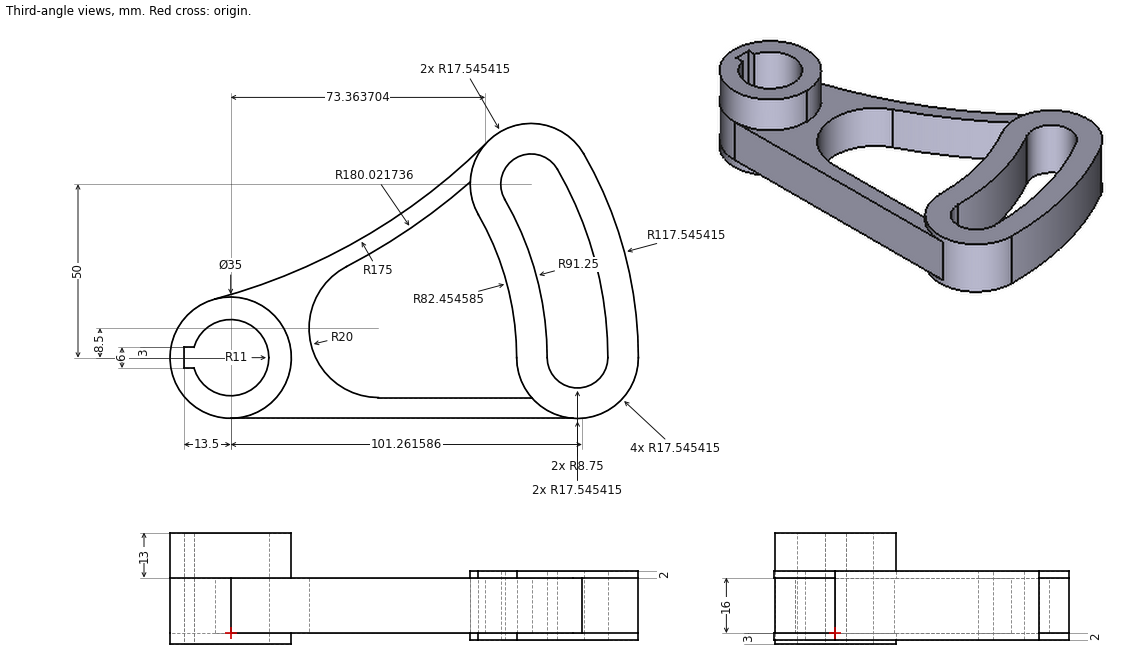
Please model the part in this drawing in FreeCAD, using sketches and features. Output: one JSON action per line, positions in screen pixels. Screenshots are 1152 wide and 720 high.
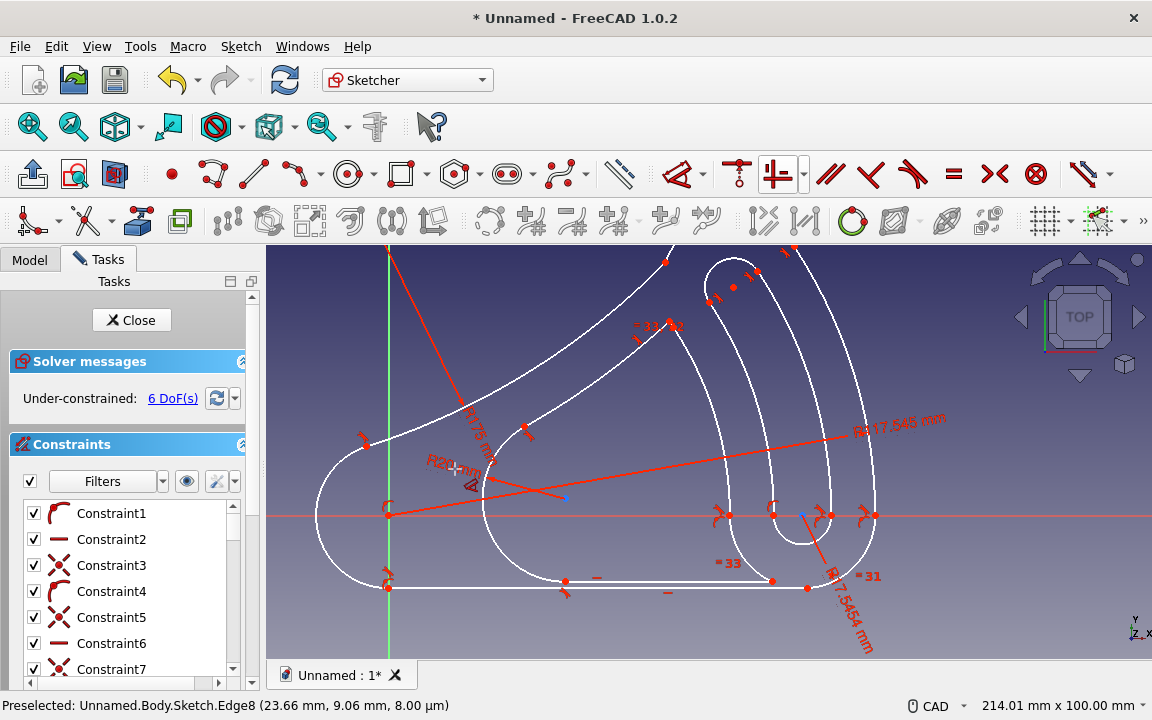
{"action": "left_click", "coordinate": [571, 399]}
{"action": "left_click", "coordinate": [589, 426]}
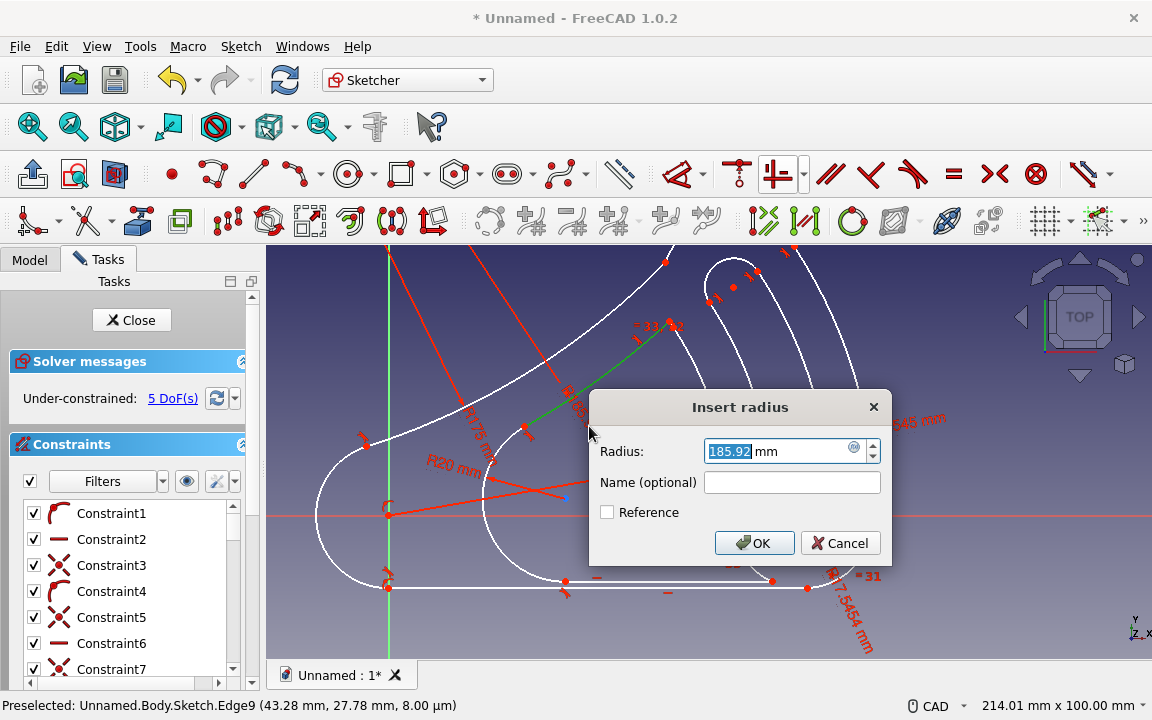
{"action": "type", "text": "180.021736"}
{"action": "key", "text": "Return"}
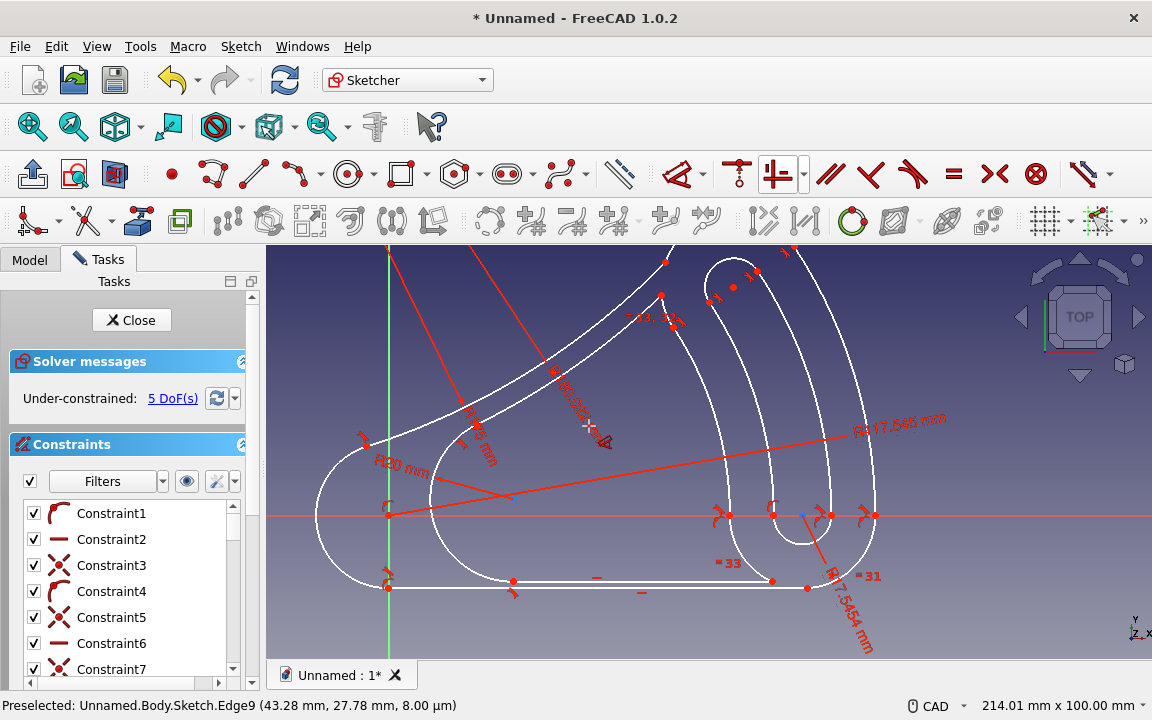
{"action": "left_click", "coordinate": [707, 277]}
{"action": "left_click", "coordinate": [712, 344]}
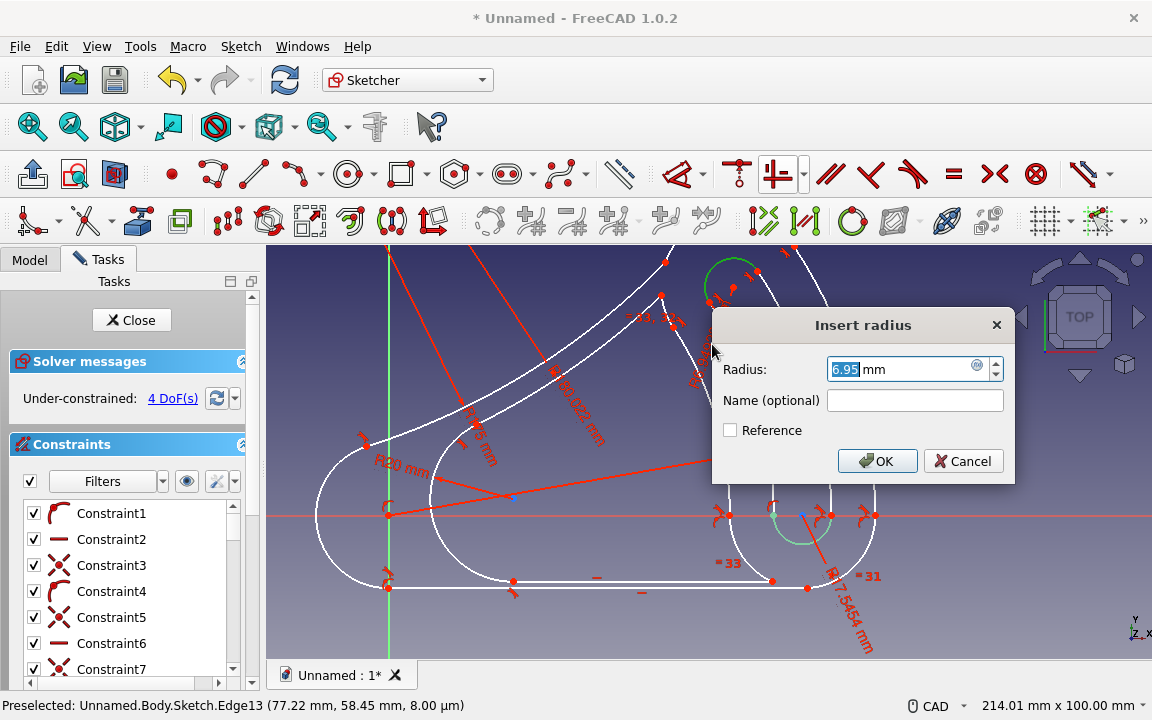
{"action": "type", "text": "8.75"}
{"action": "key", "text": "Return"}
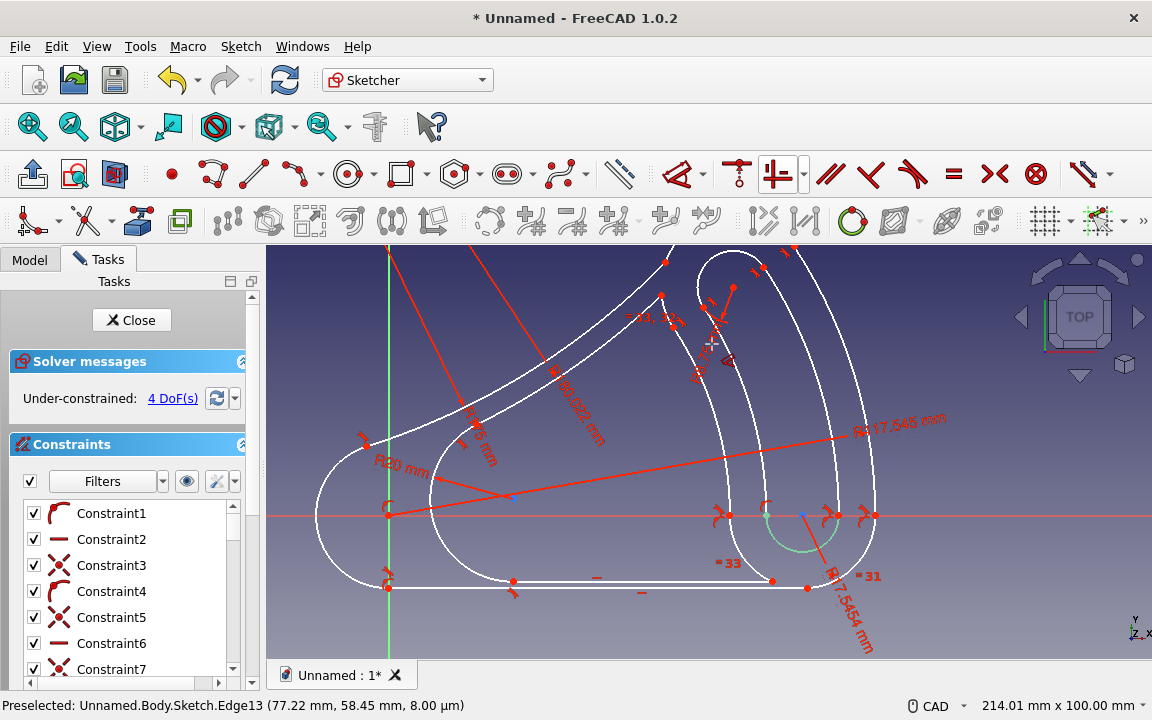
{"action": "left_click", "coordinate": [734, 287]}
{"action": "left_click", "coordinate": [355, 401]}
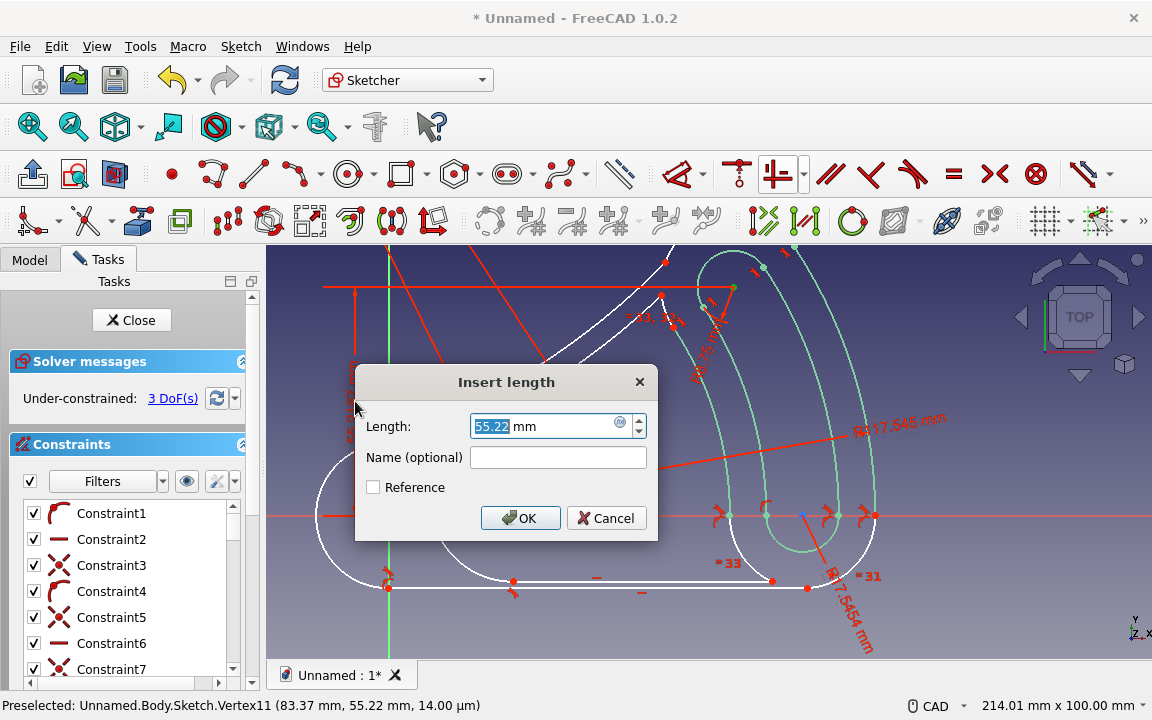
{"action": "type", "text": "50"}
{"action": "key", "text": "Return"}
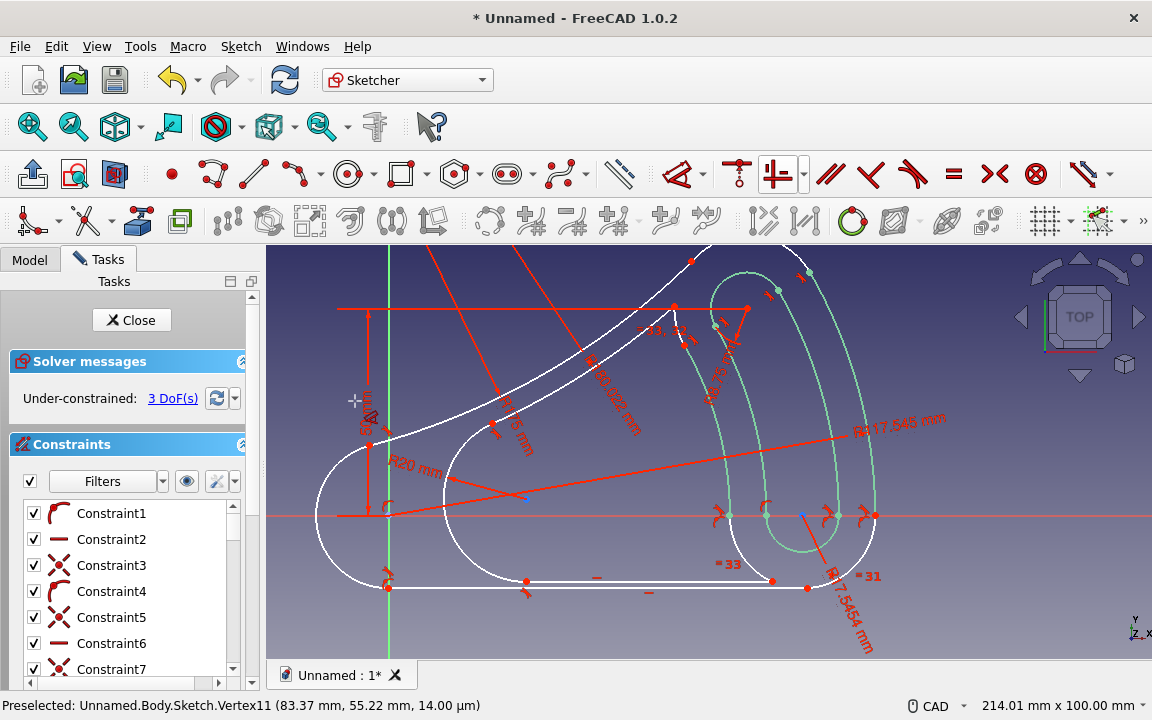
{"action": "left_click", "coordinate": [527, 499]}
{"action": "left_click", "coordinate": [355, 502]}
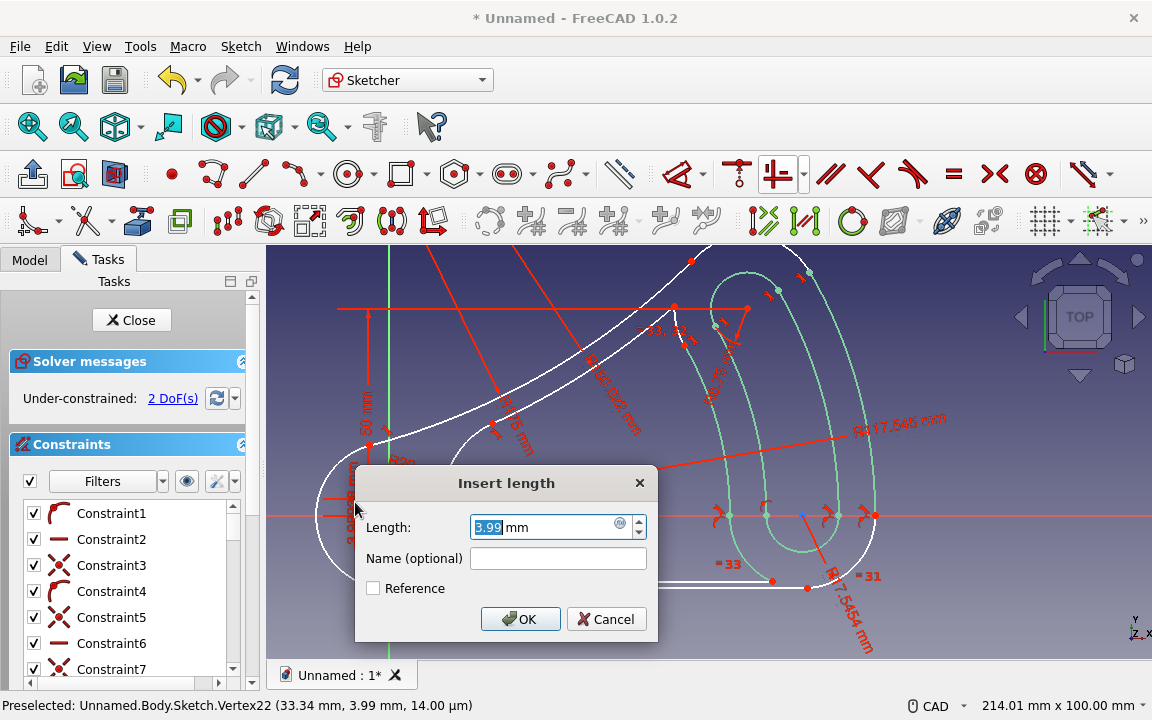
{"action": "type", "text": "8.5"}
{"action": "key", "text": "Return"}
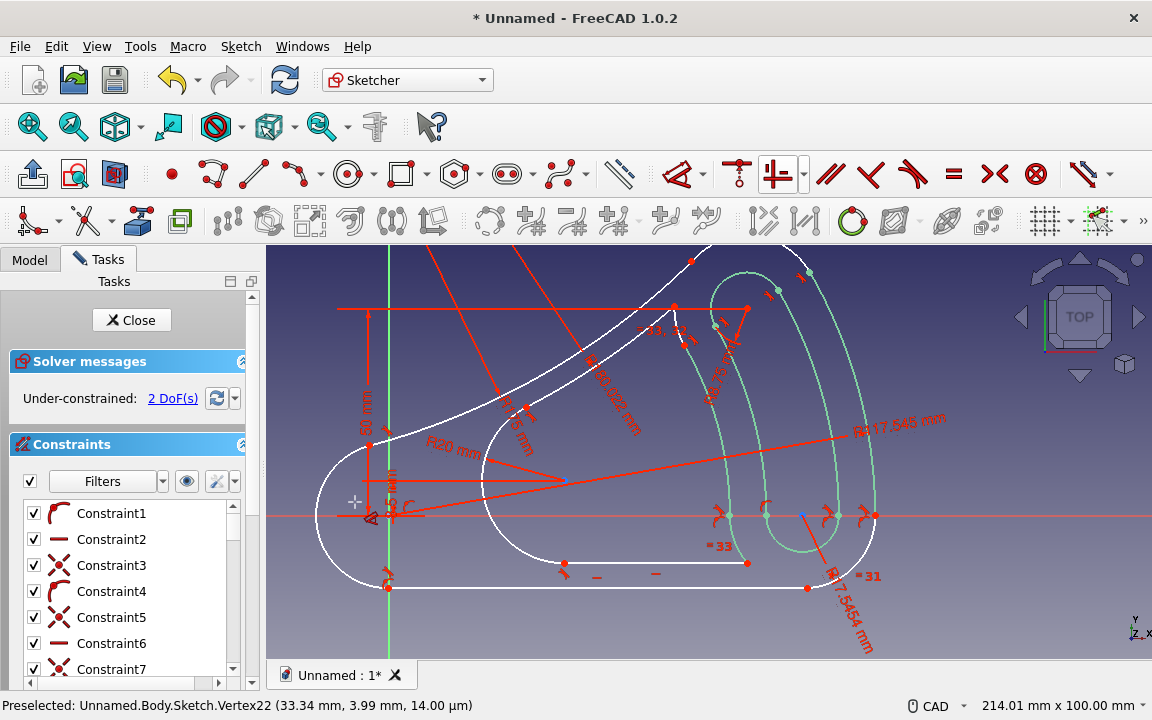
{"action": "left_click", "coordinate": [514, 588]}
{"action": "left_click", "coordinate": [598, 622]}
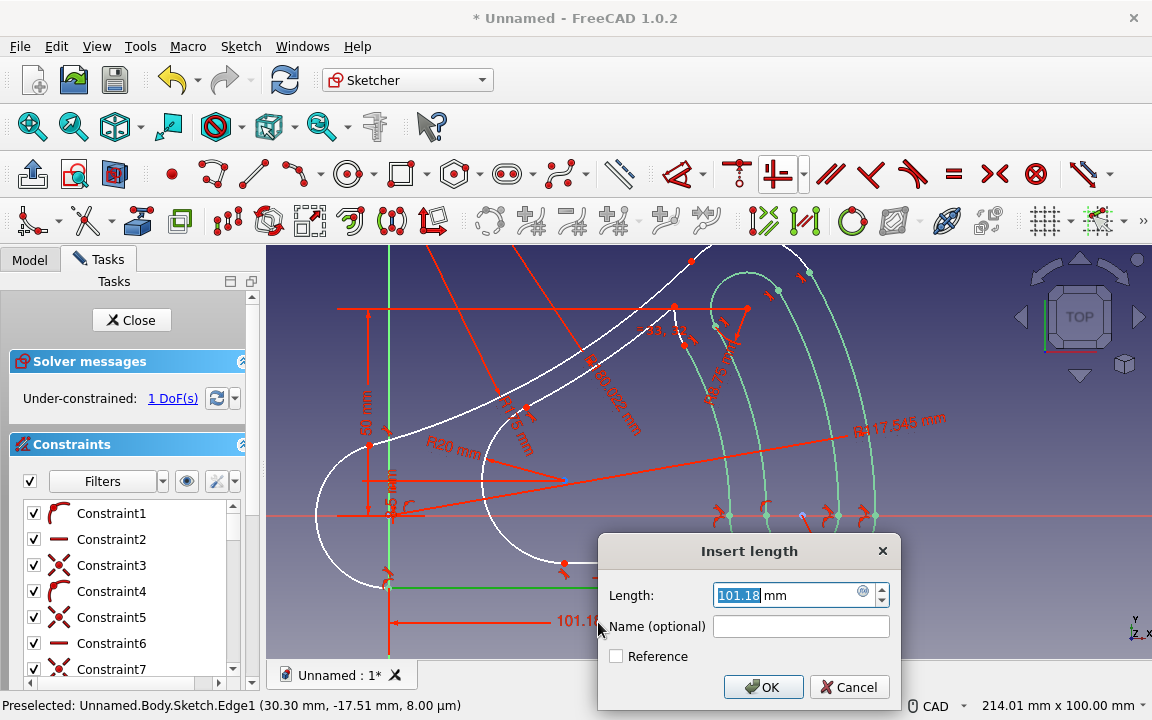
{"action": "type", "text": "101.261586"}
{"action": "key", "text": "Return"}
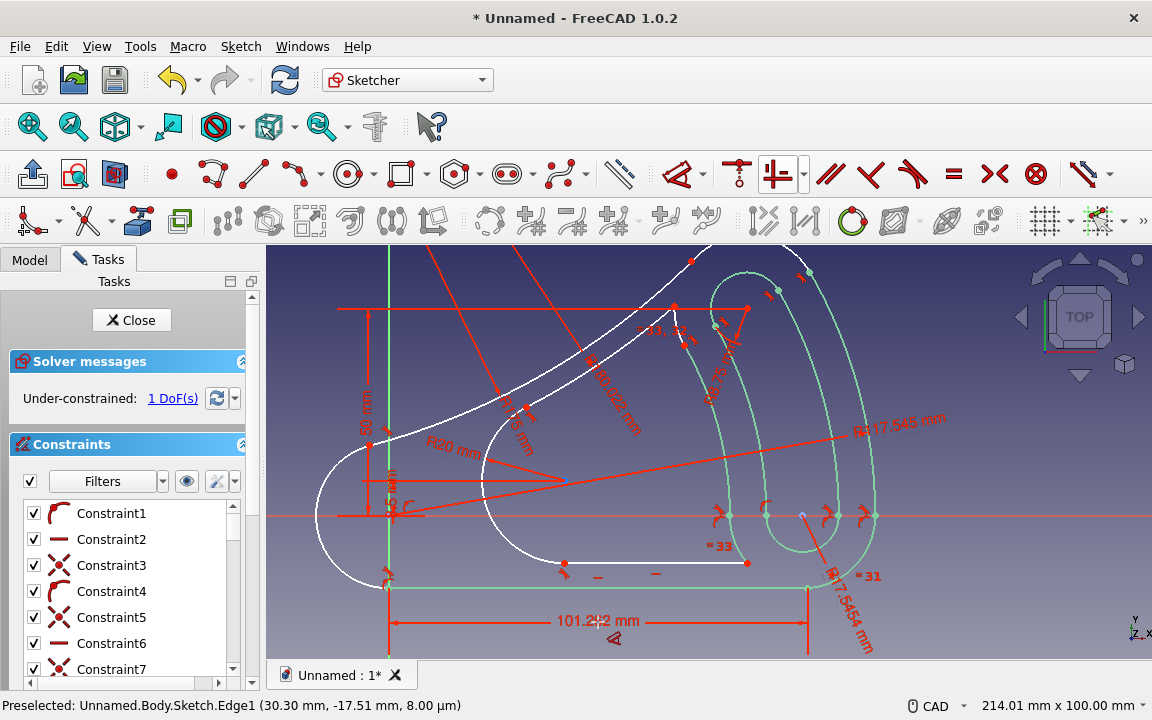
{"action": "scroll", "coordinate": [731, 533], "scroll_direction": "down", "scroll_amount": 2}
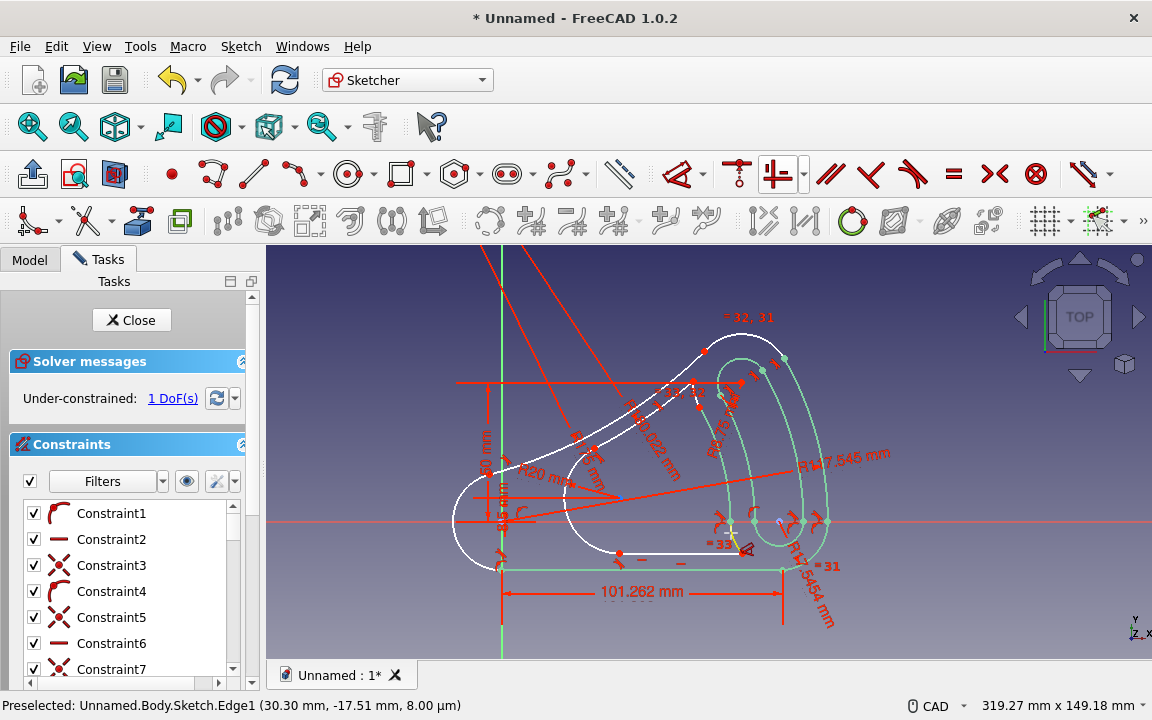
{"action": "left_click", "coordinate": [705, 351]}
{"action": "left_click", "coordinate": [603, 317]}